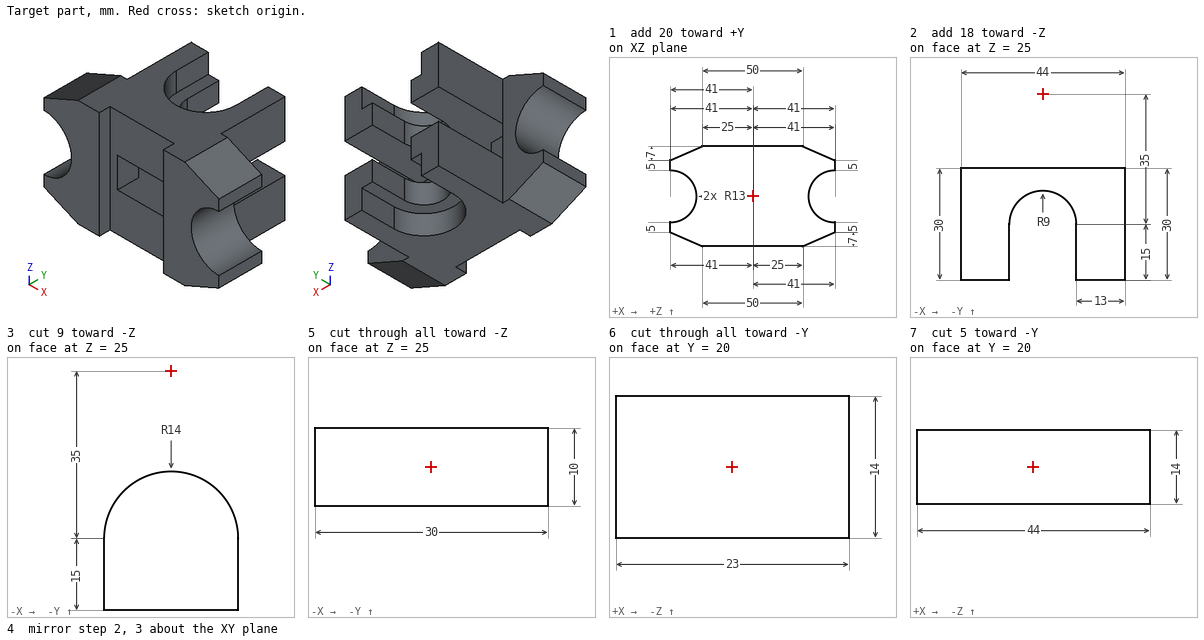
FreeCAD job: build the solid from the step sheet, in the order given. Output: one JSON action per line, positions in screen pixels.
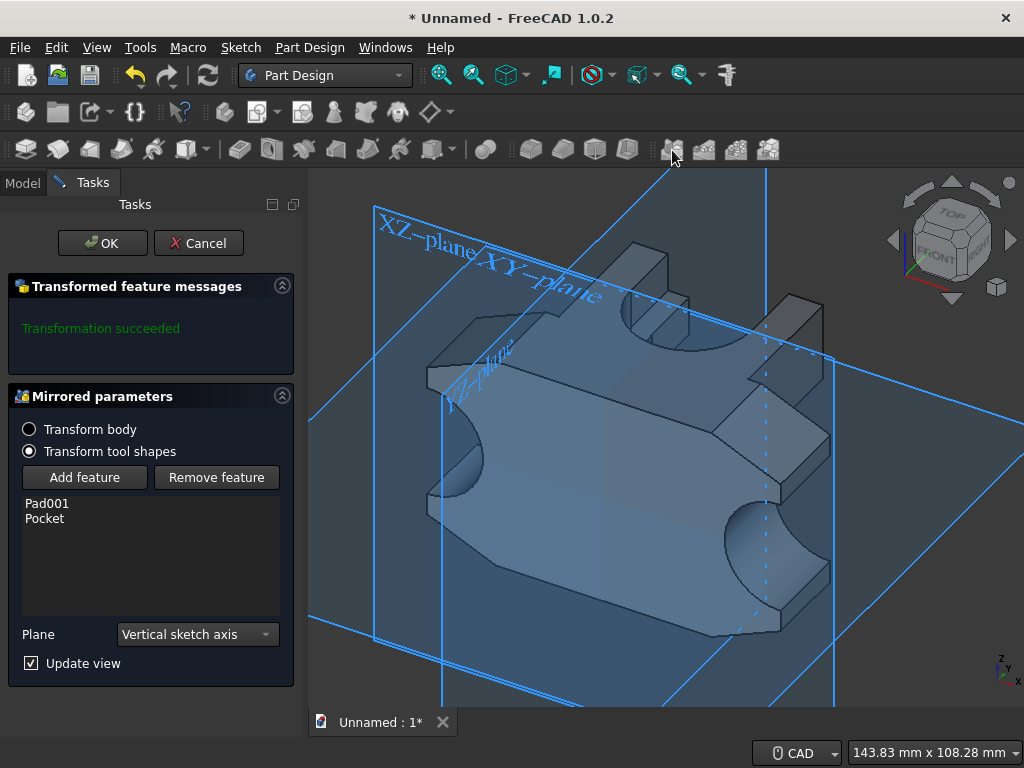
{"action": "left_click", "coordinate": [198, 634]}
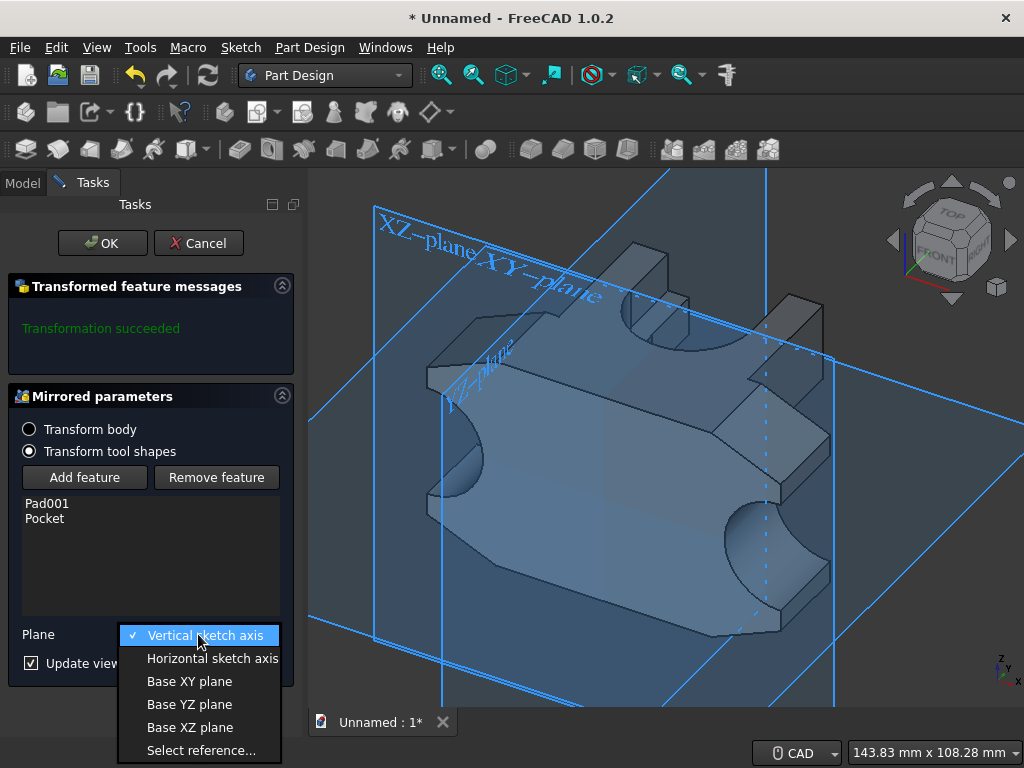
{"action": "left_click", "coordinate": [198, 682]}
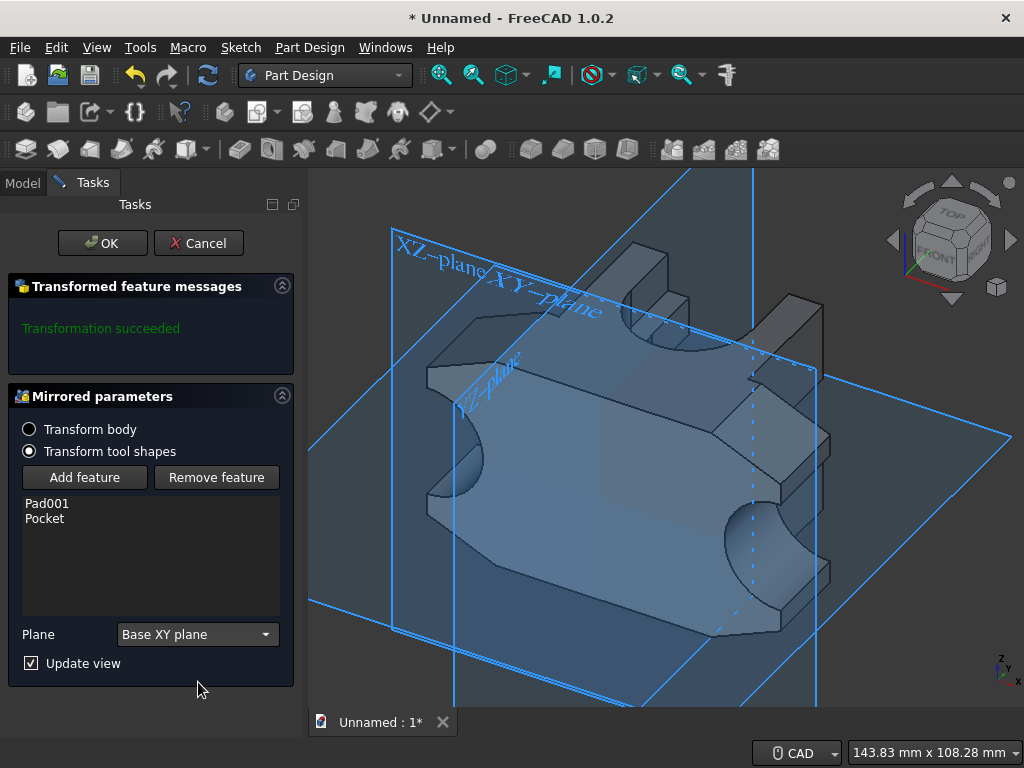
{"action": "left_click", "coordinate": [103, 243]}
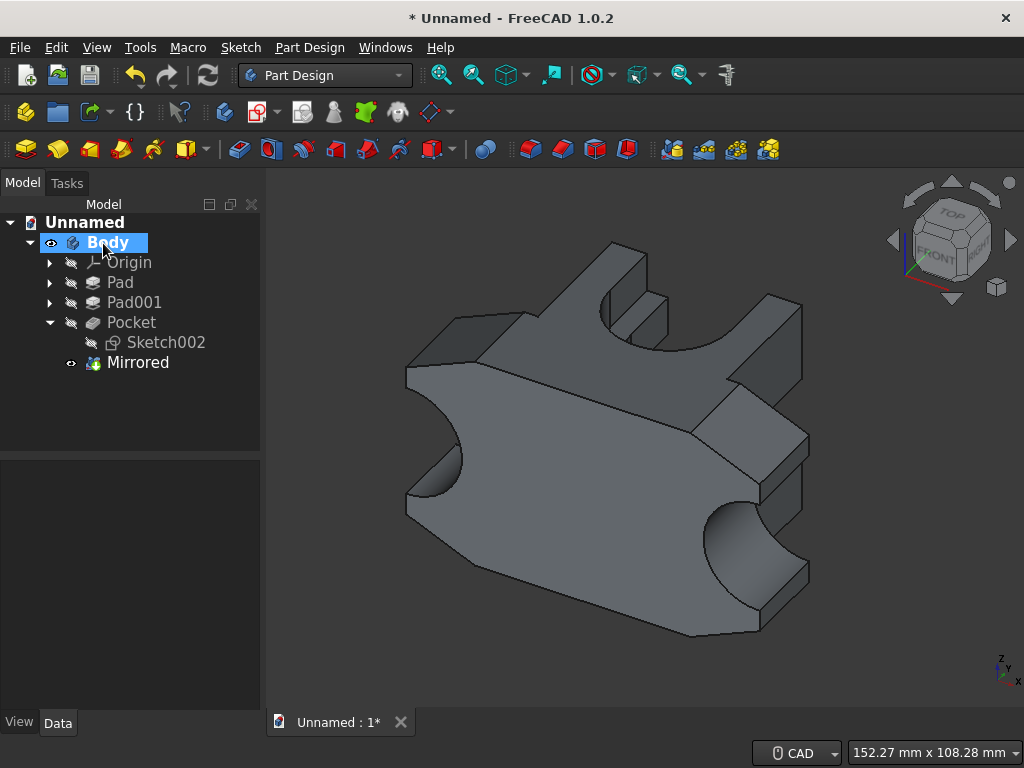
{"action": "left_click", "coordinate": [671, 390]}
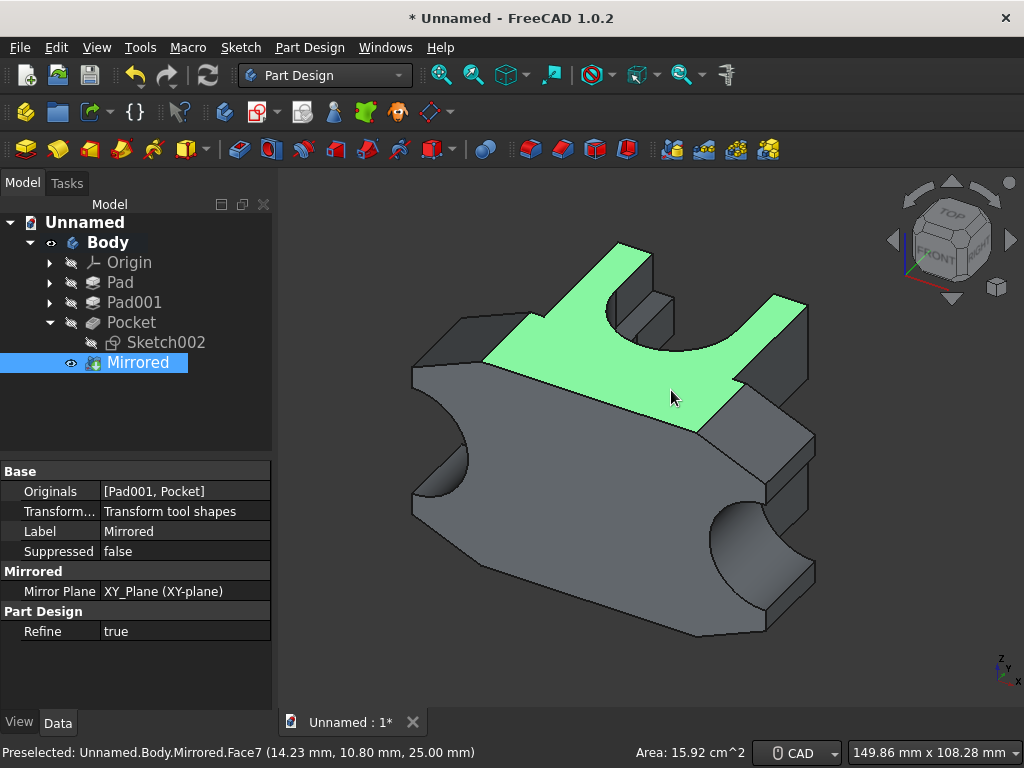
{"action": "left_click", "coordinate": [258, 112]}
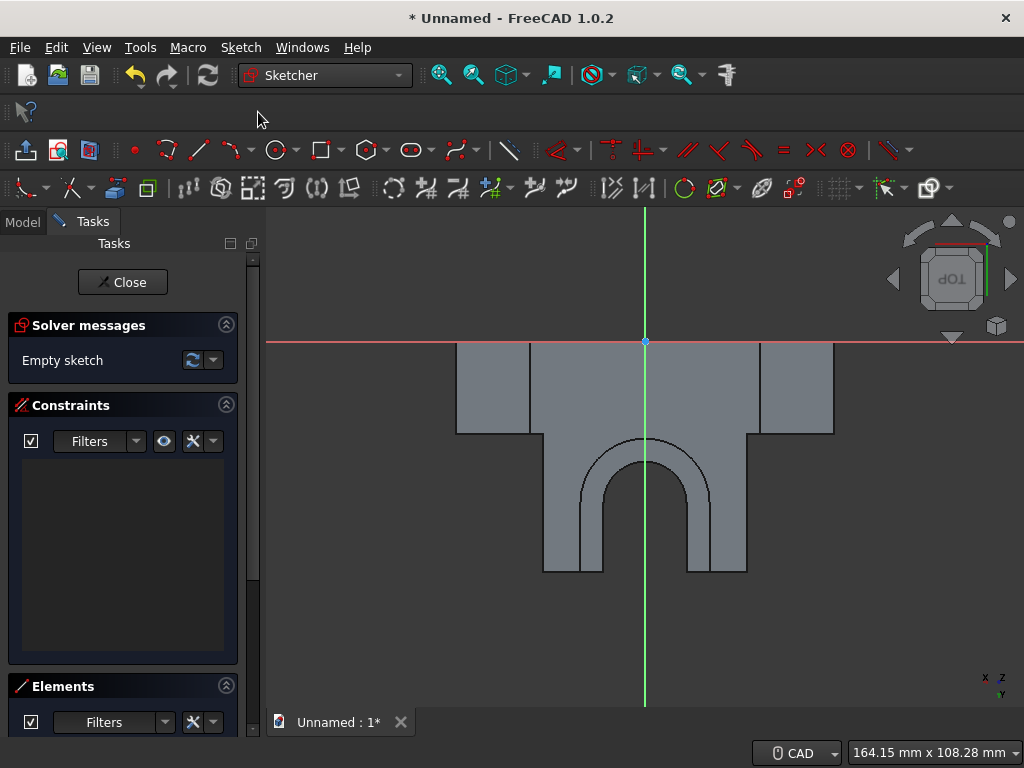
{"action": "scroll", "coordinate": [685, 274], "scroll_direction": "up", "scroll_amount": 5}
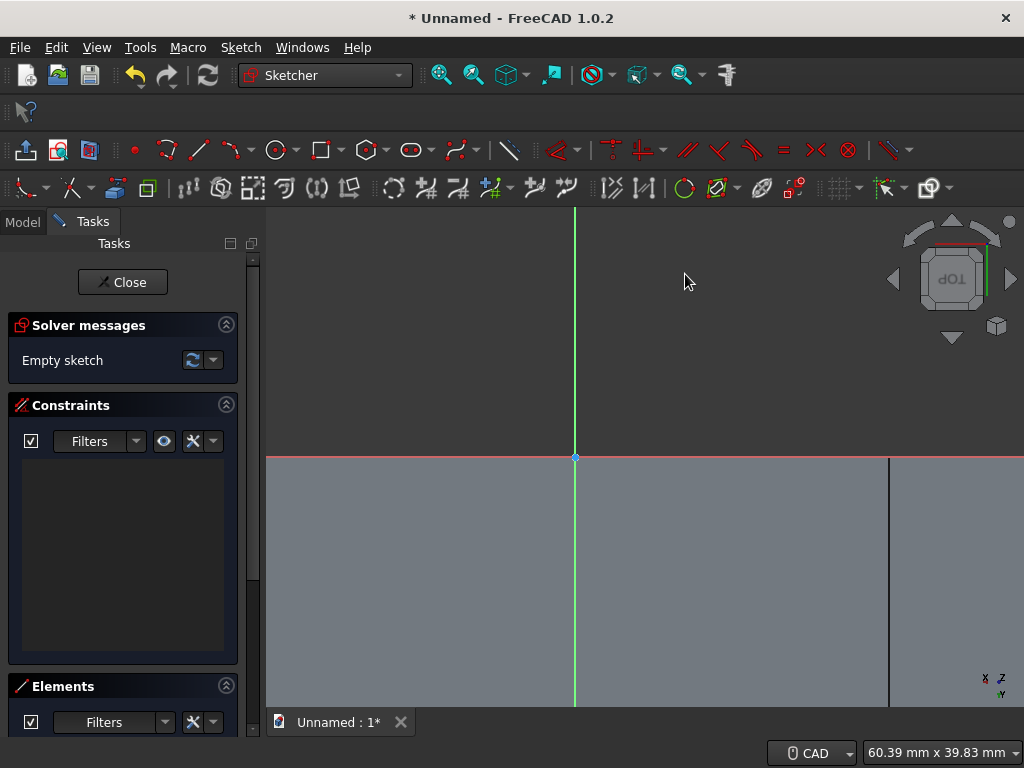
{"action": "key", "text": "g v"}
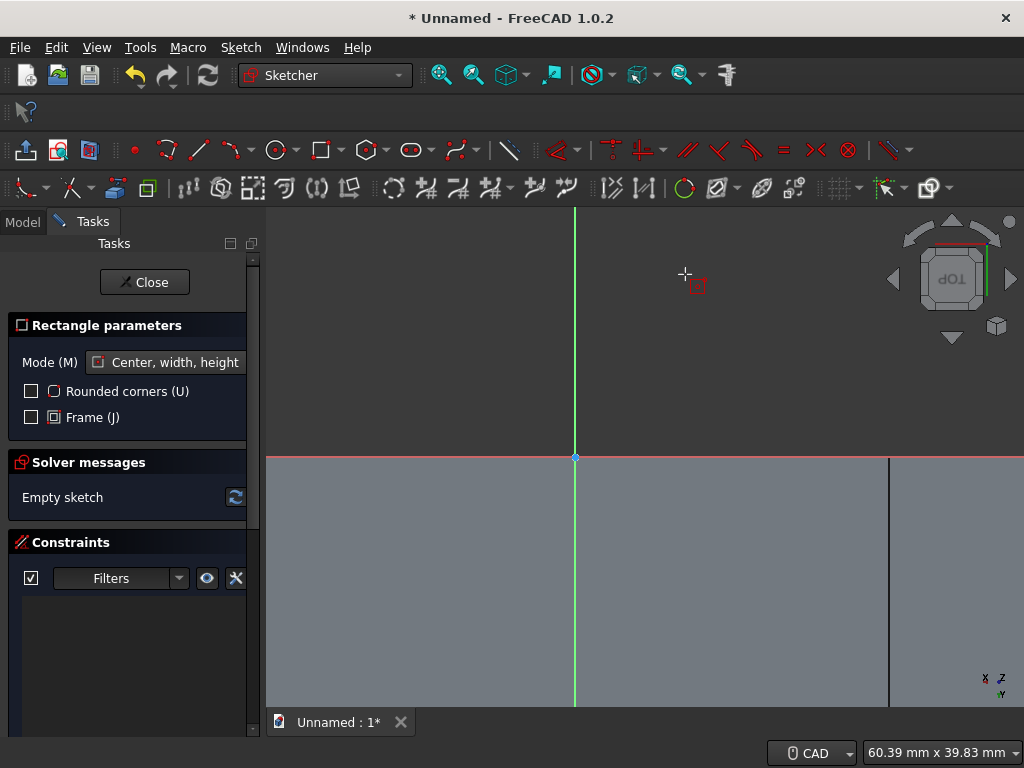
{"action": "left_click", "coordinate": [575, 457]}
{"action": "mouse_move", "coordinate": [764, 395]}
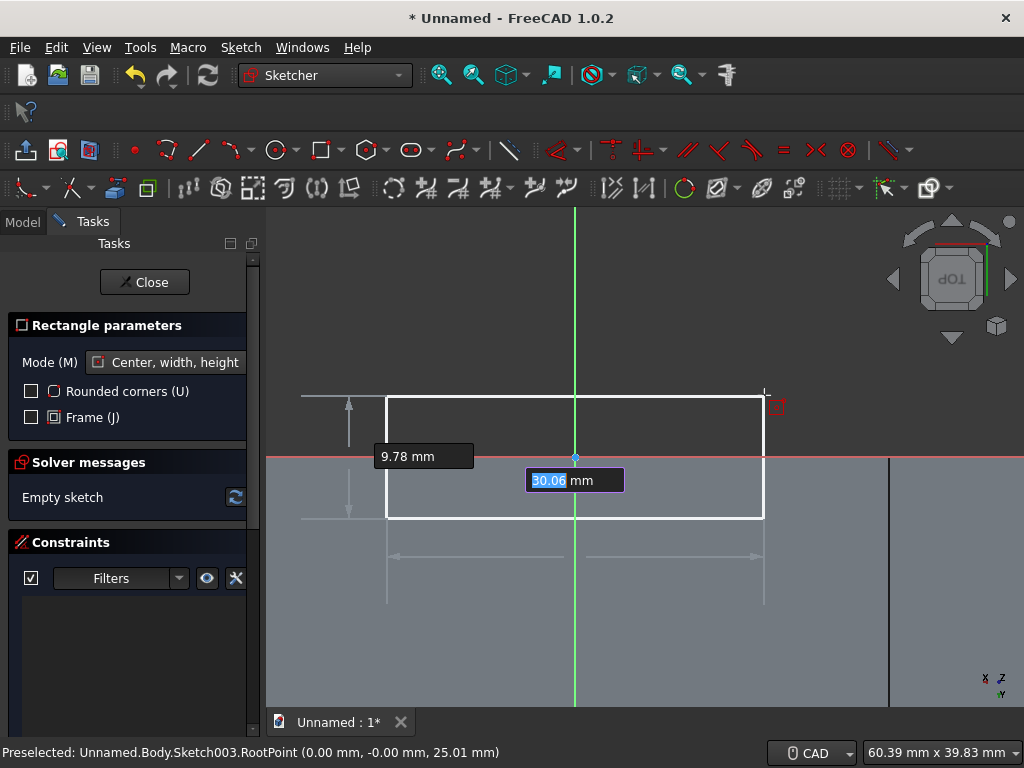
{"action": "type", "text": "30"}
{"action": "key", "text": "Tab"}
{"action": "type", "text": "10"}
{"action": "key", "text": "Return"}
{"action": "key", "text": "Escape"}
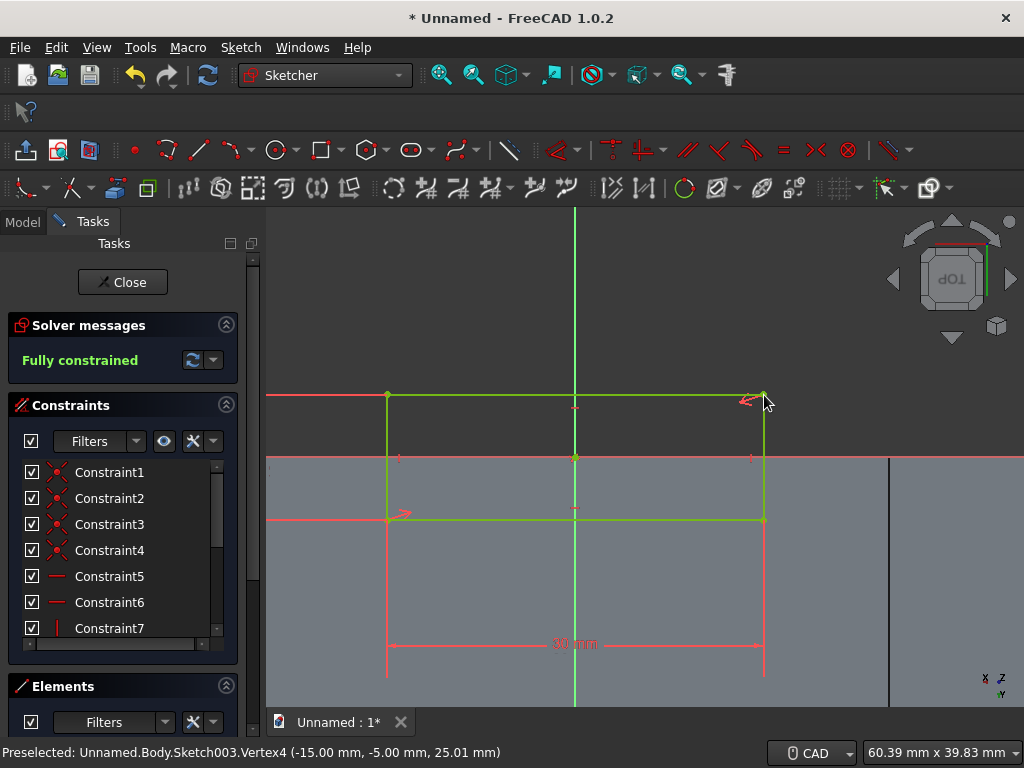
{"action": "left_click", "coordinate": [123, 282]}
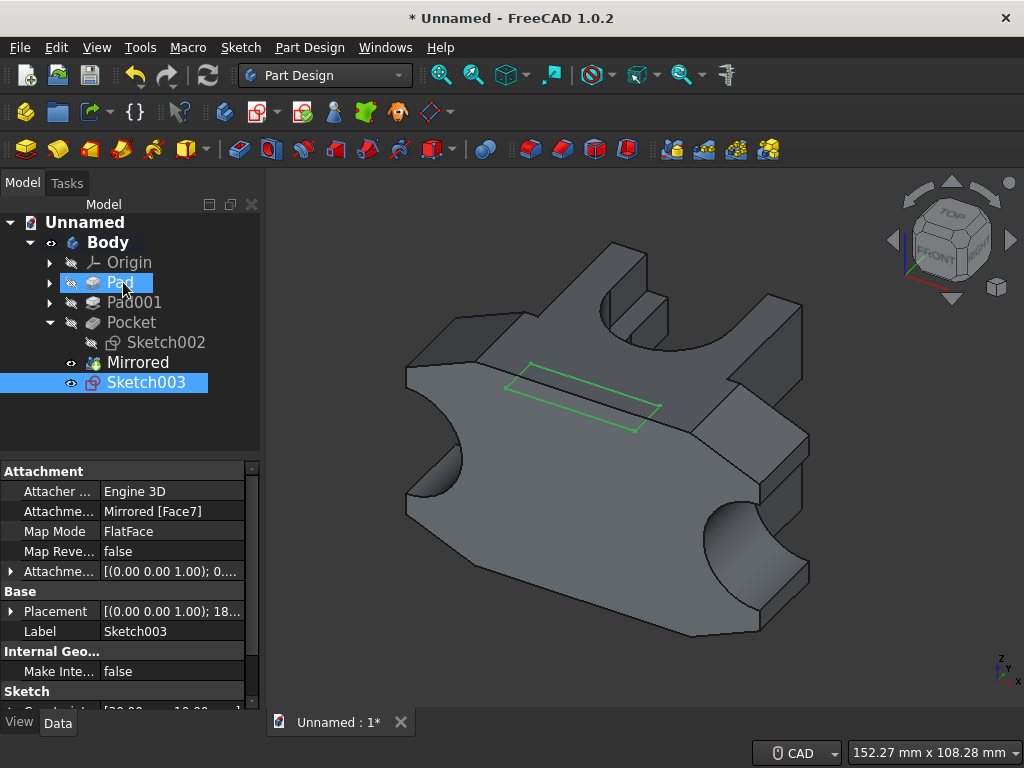
{"action": "left_click", "coordinate": [240, 150]}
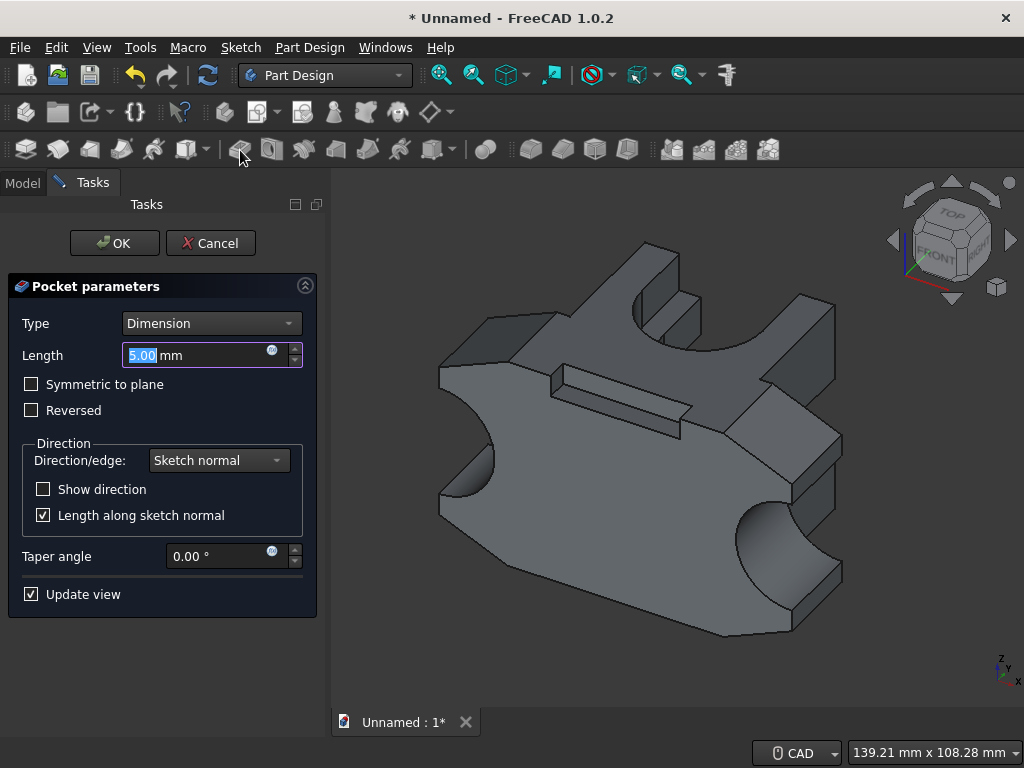
{"action": "left_click", "coordinate": [212, 324]}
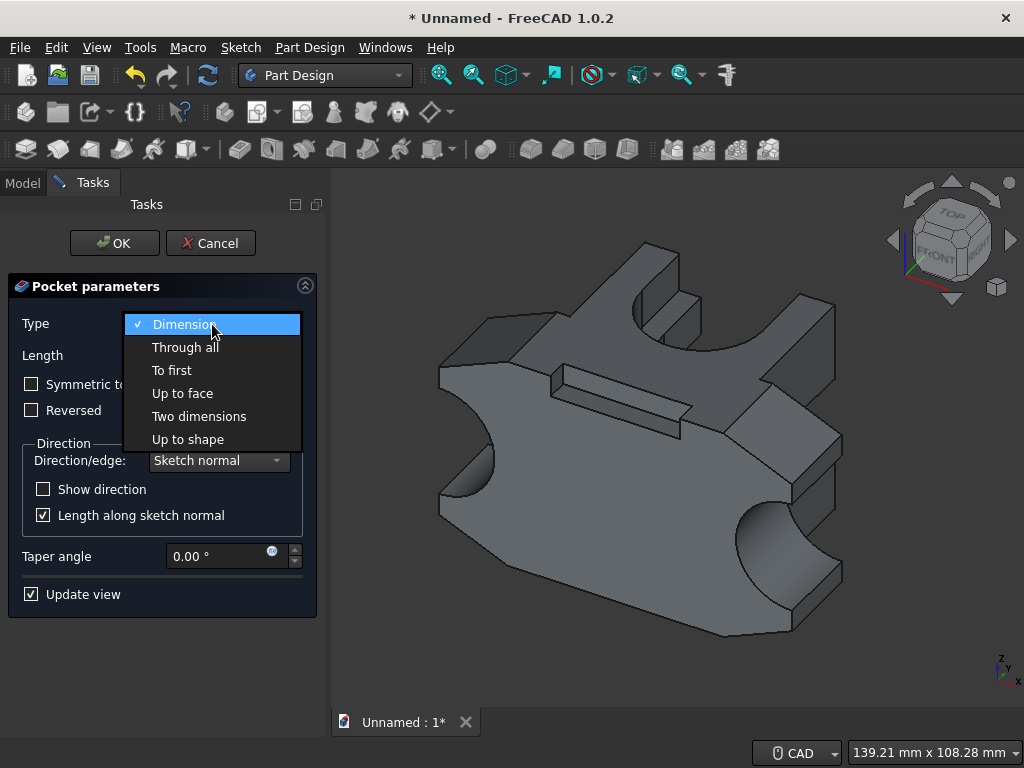
{"action": "left_click", "coordinate": [212, 348]}